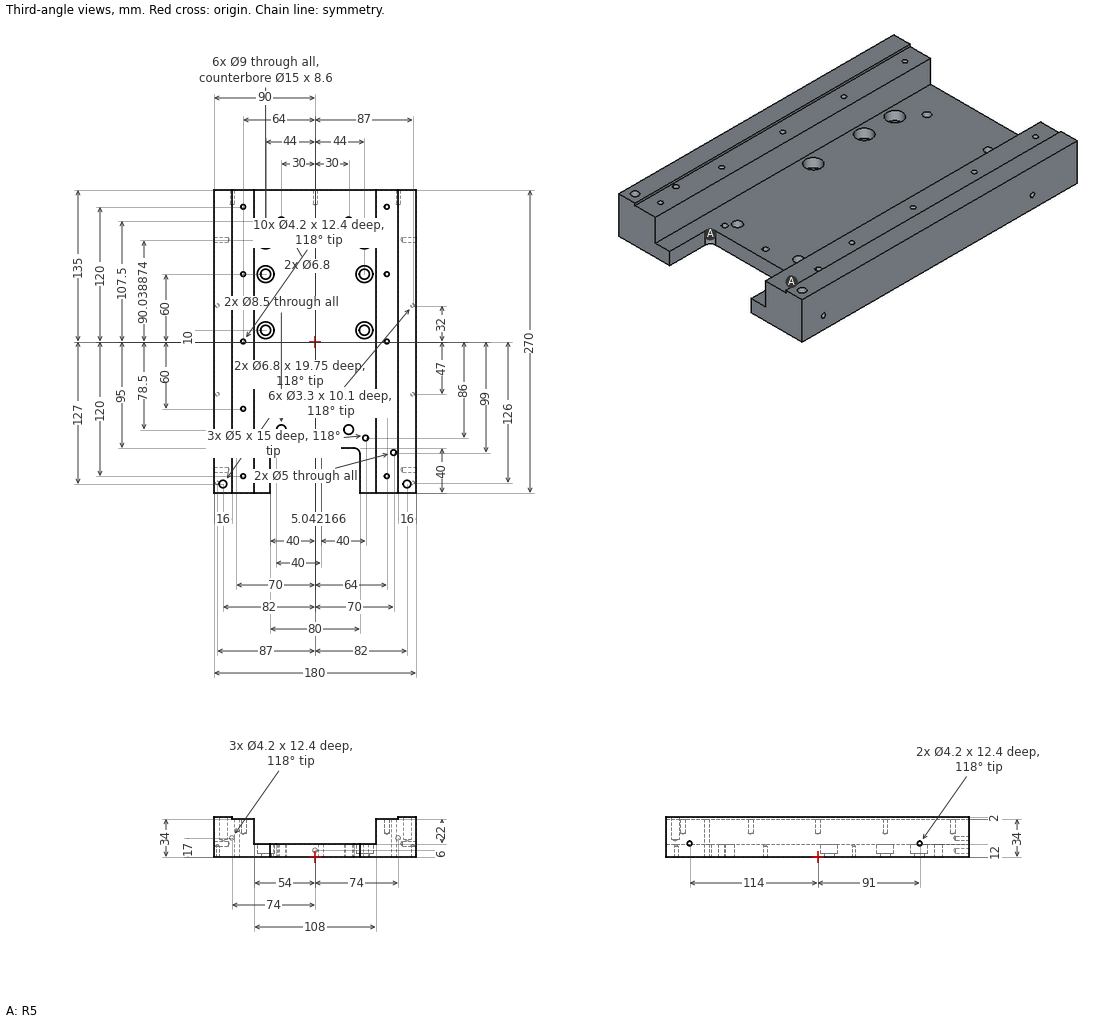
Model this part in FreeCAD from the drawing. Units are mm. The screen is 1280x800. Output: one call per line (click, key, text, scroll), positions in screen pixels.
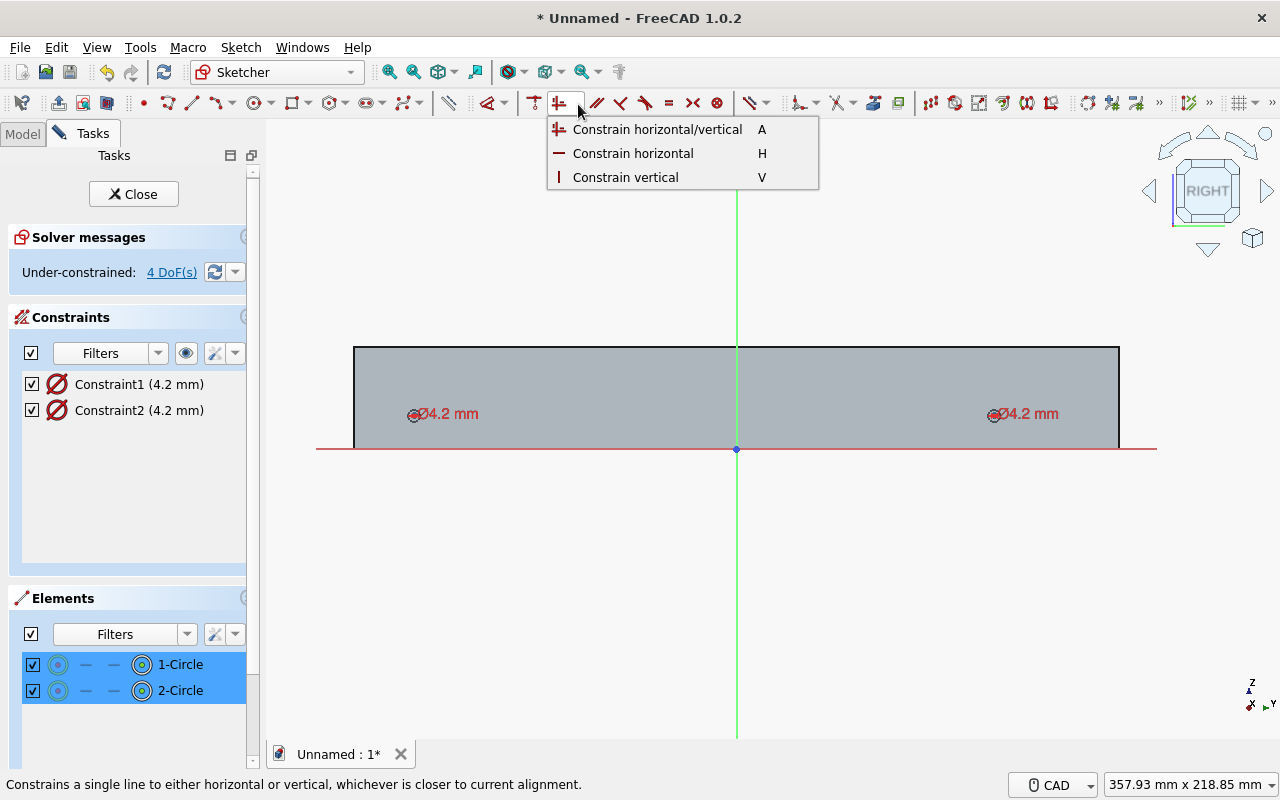
click(683, 153)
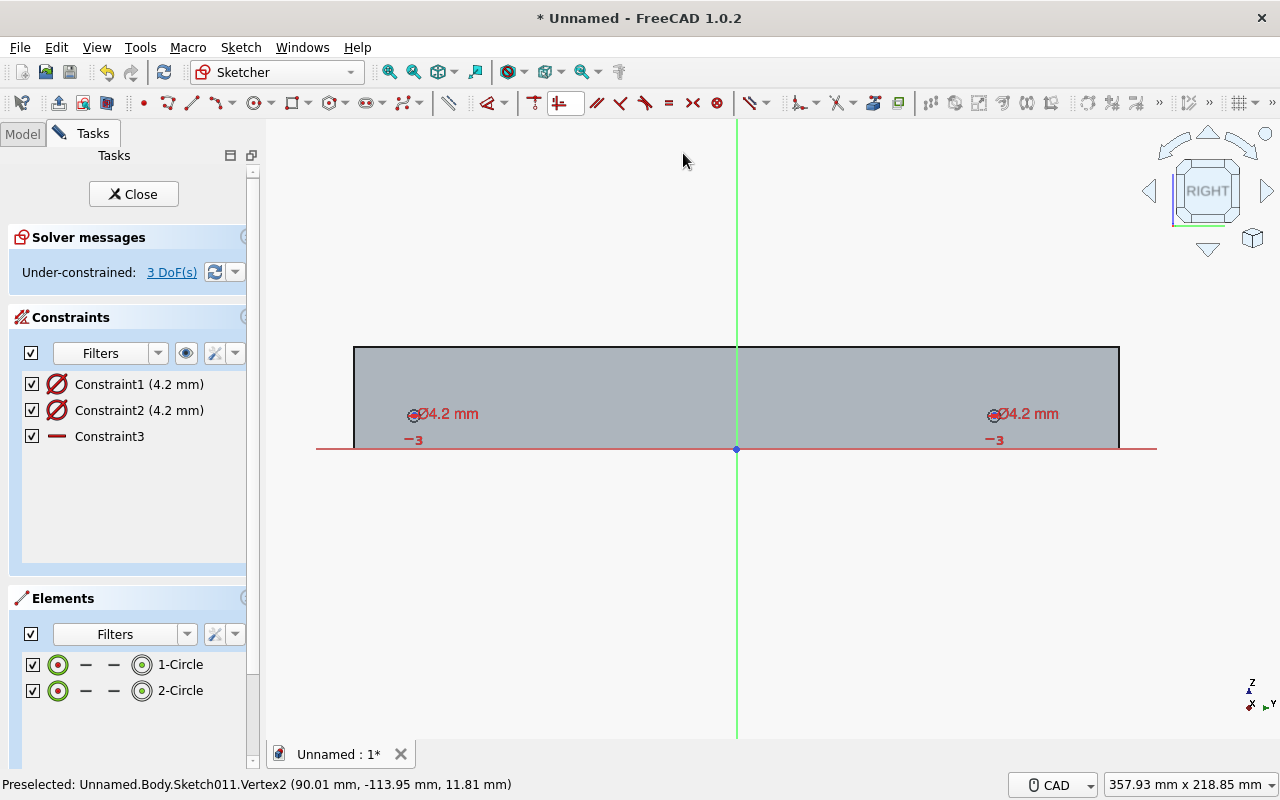
click(488, 104)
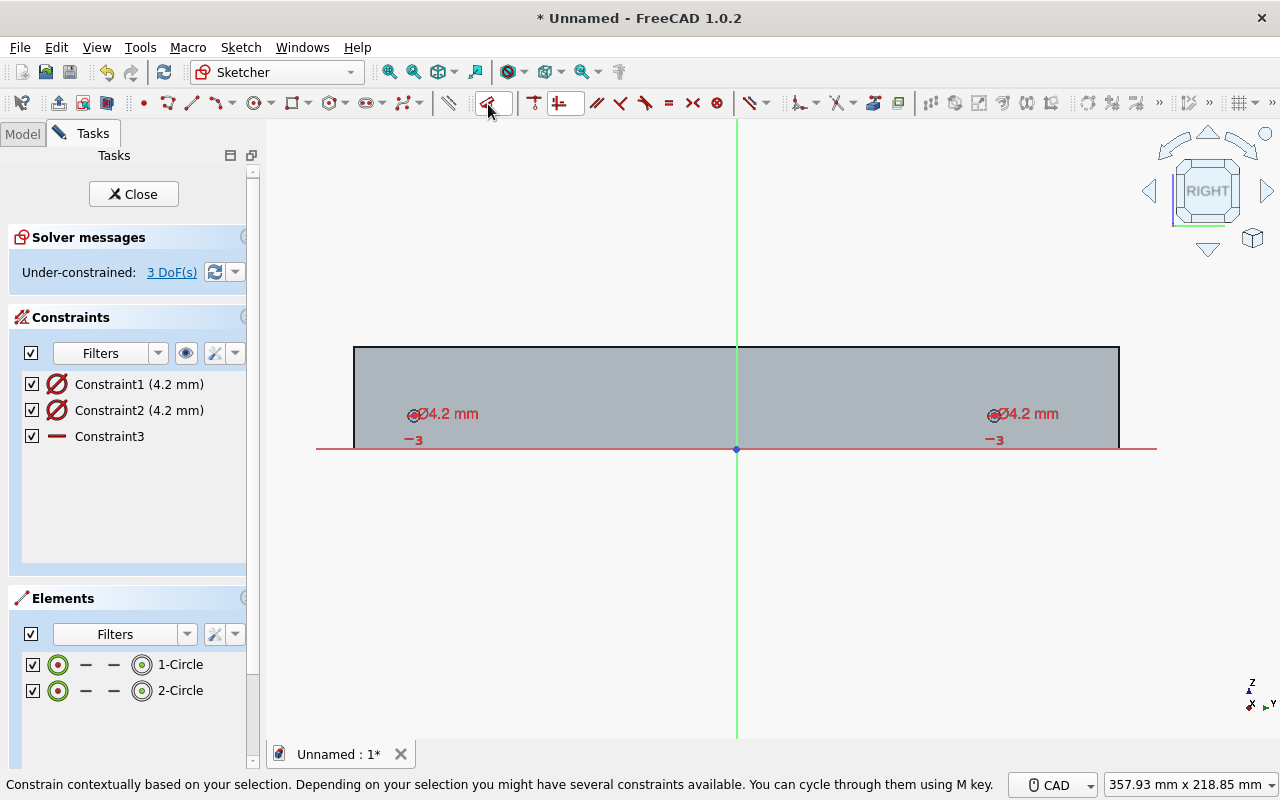
click(994, 416)
click(866, 483)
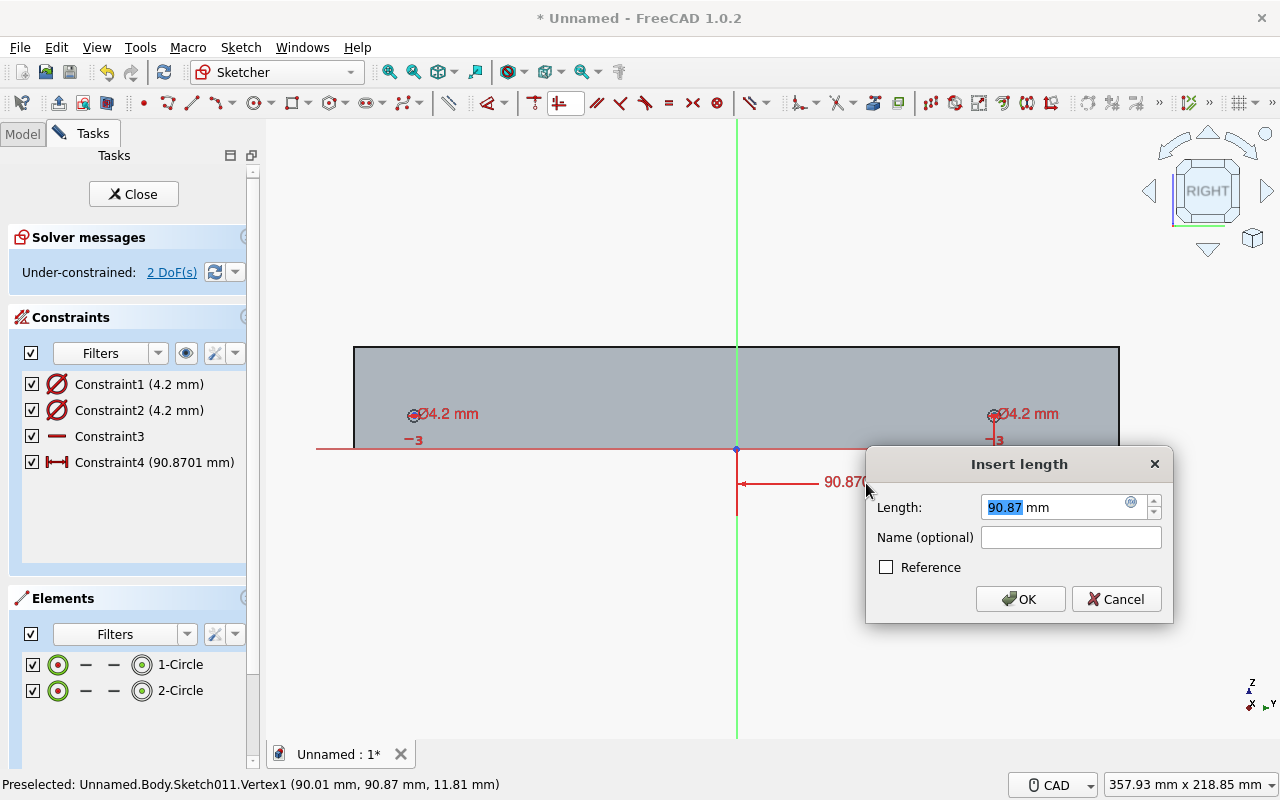
text(91)
key(Return)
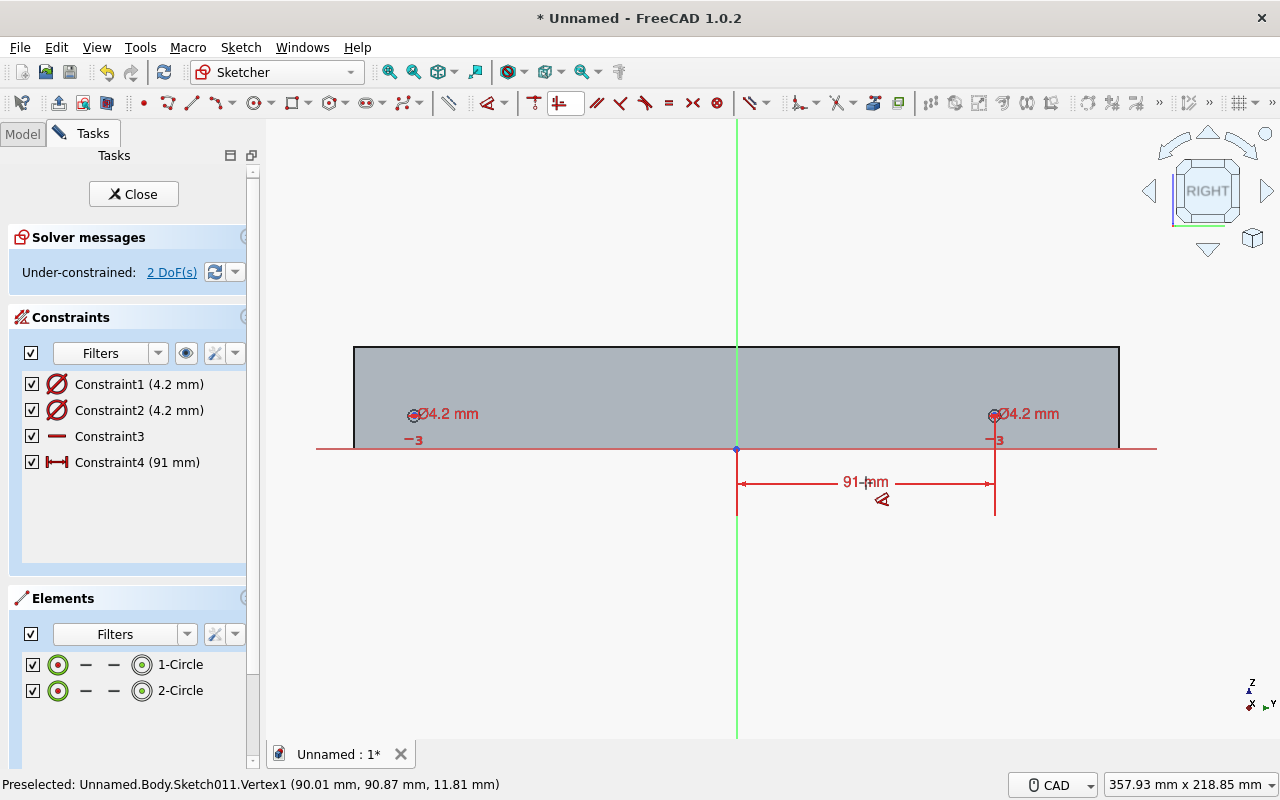
click(995, 416)
click(1029, 433)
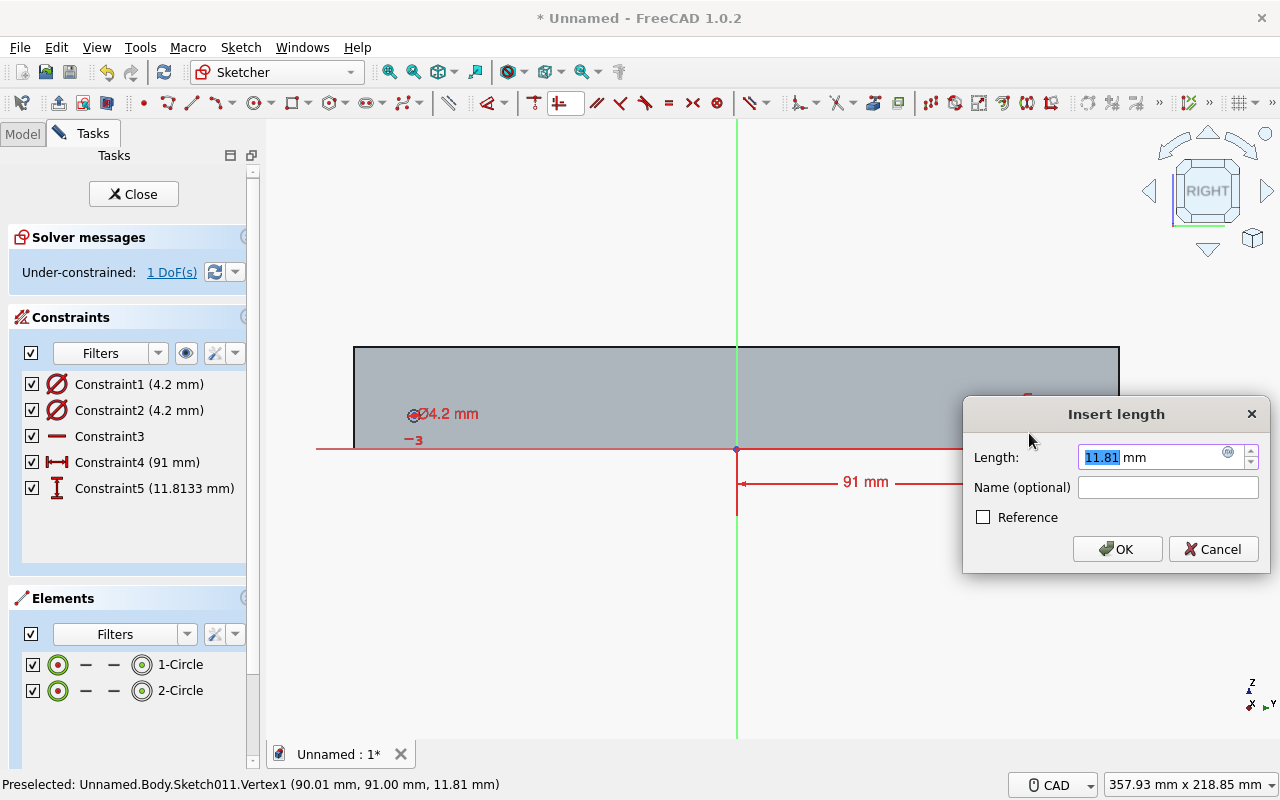
text(12)
key(Return)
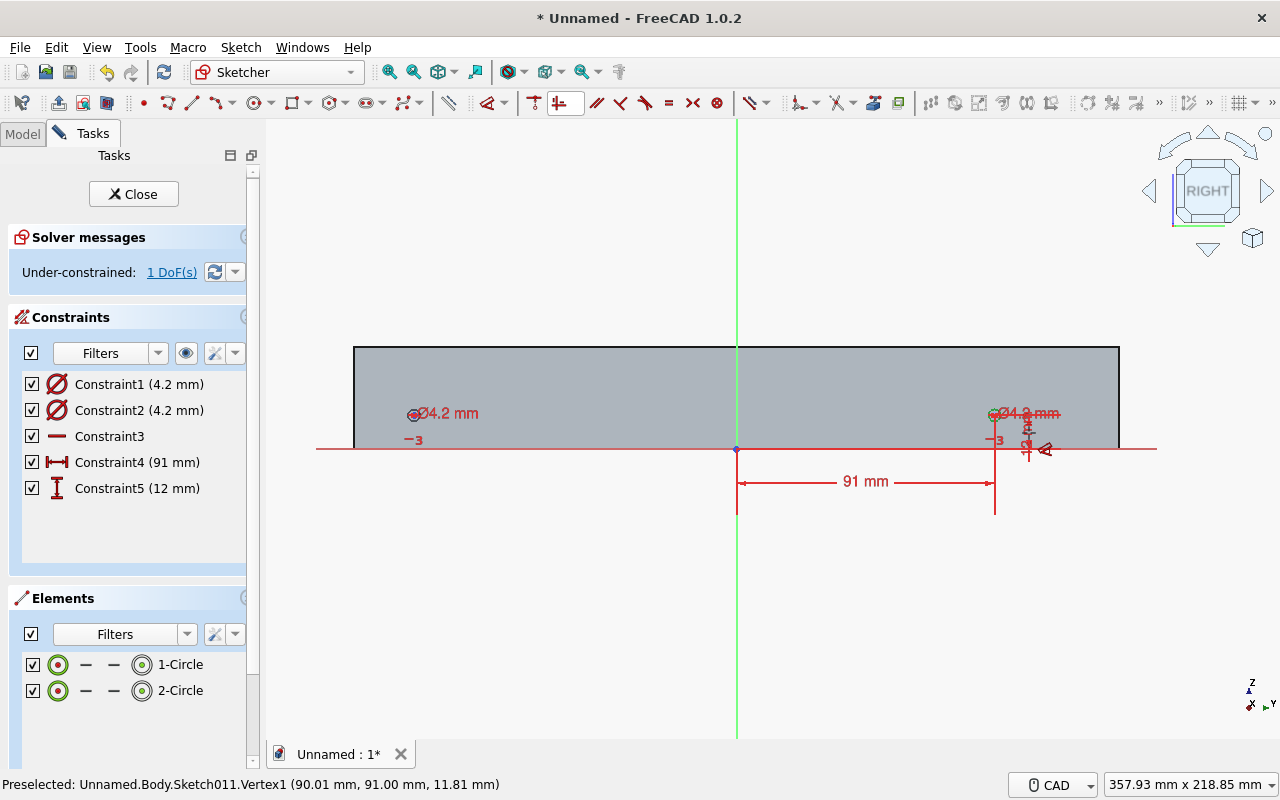
click(414, 415)
click(575, 483)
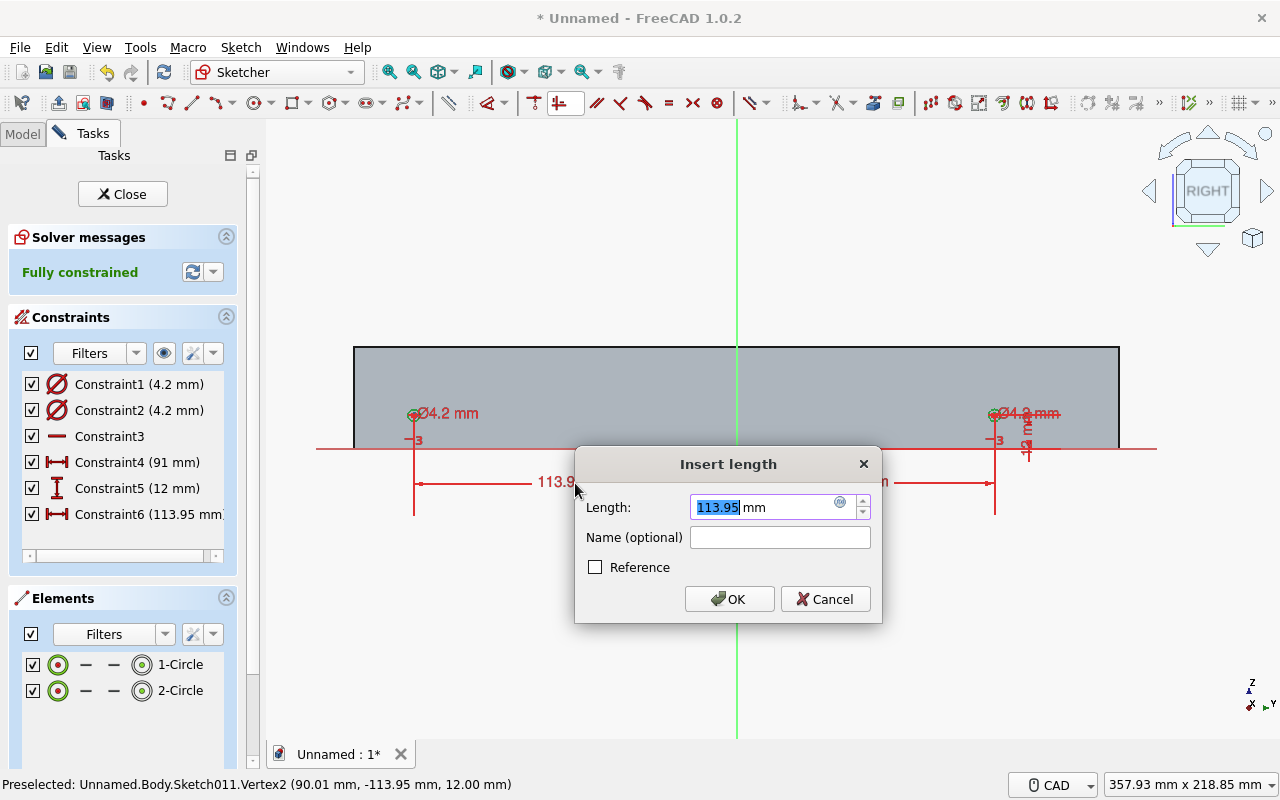
text(114)
key(Return)
key(Escape)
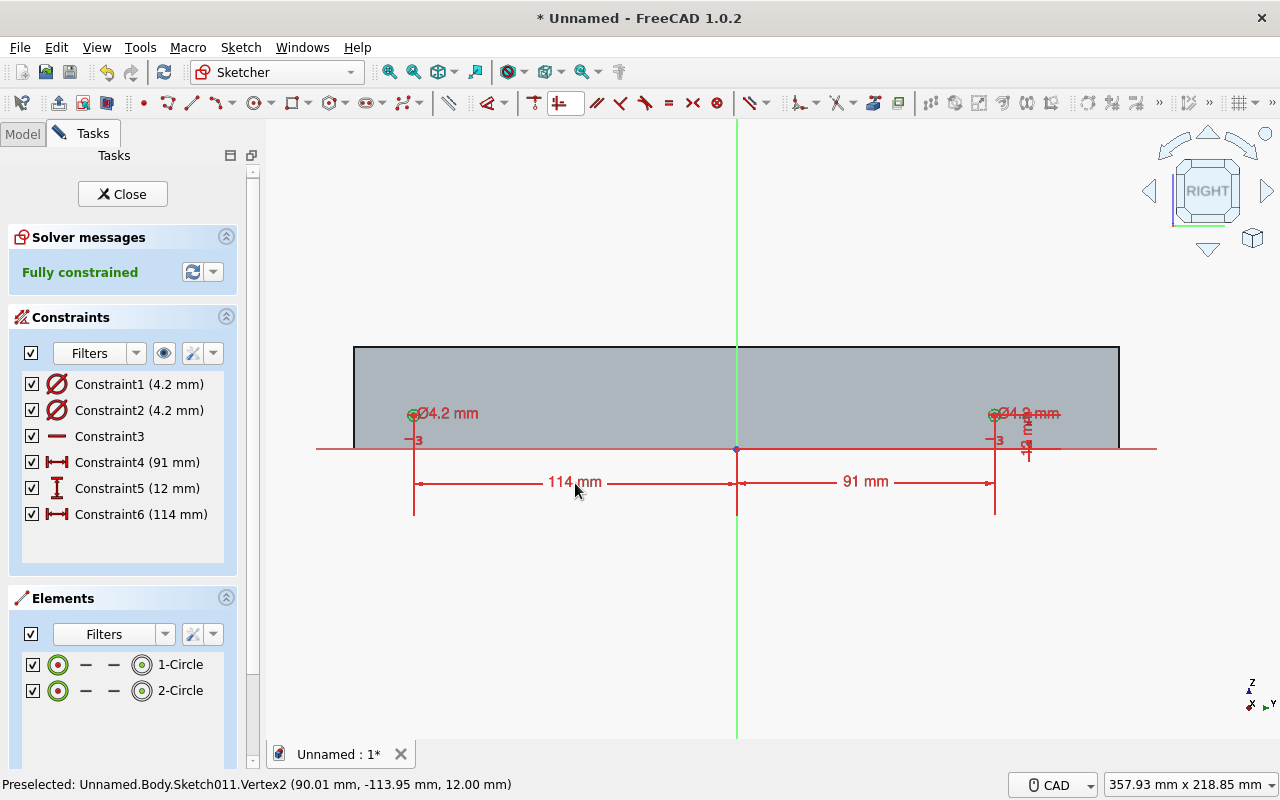
click(123, 194)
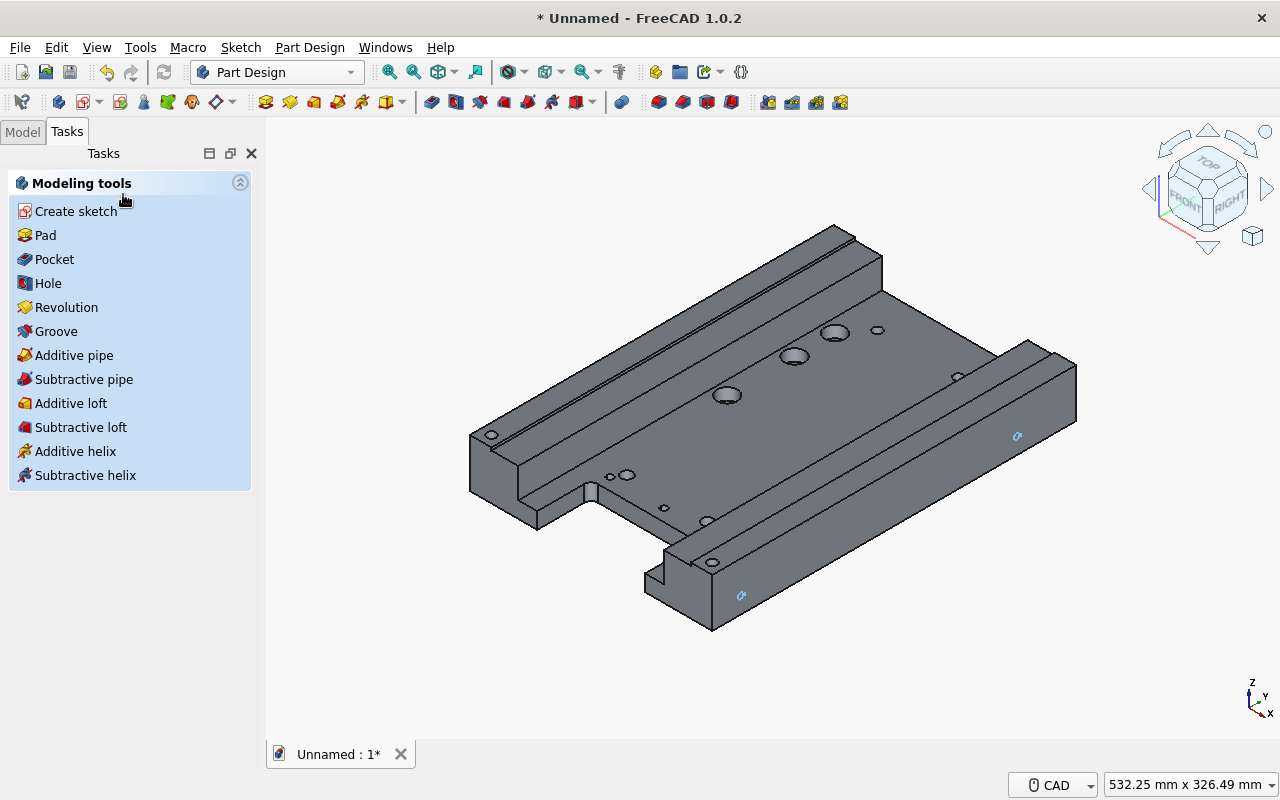
click(456, 102)